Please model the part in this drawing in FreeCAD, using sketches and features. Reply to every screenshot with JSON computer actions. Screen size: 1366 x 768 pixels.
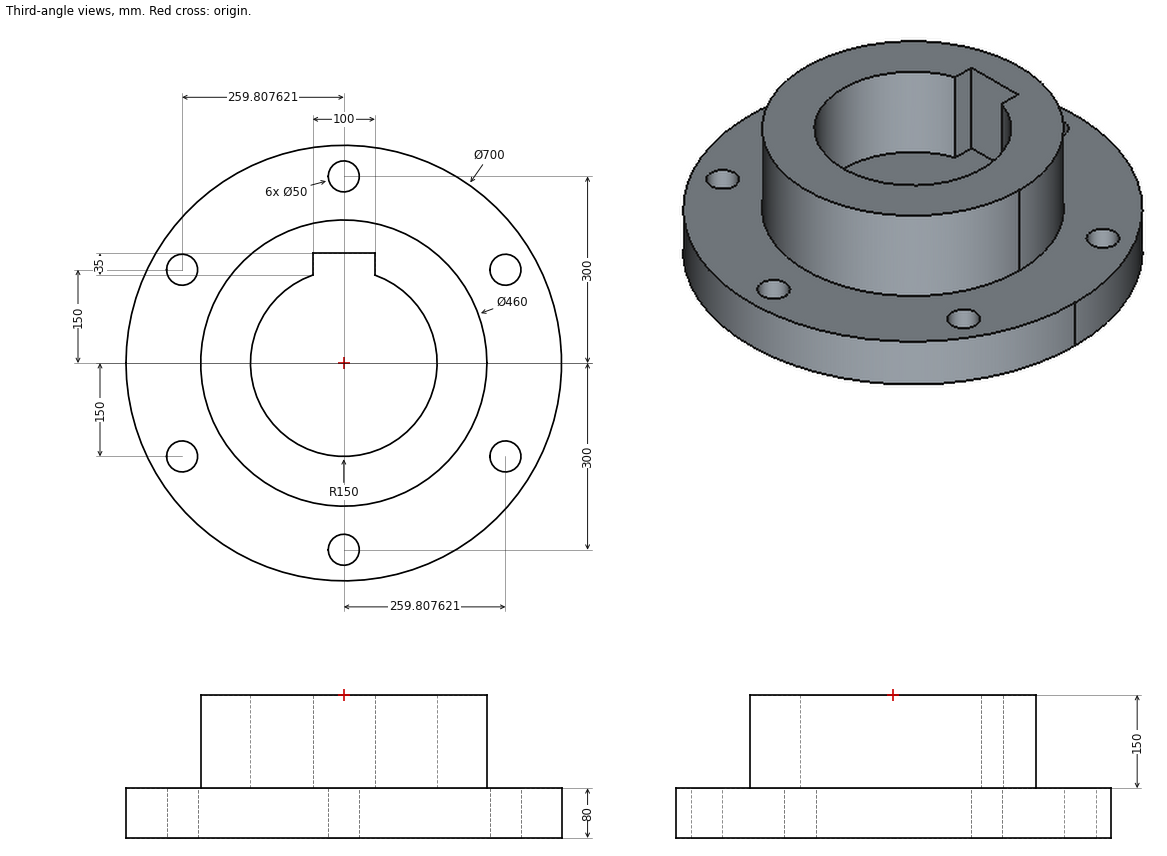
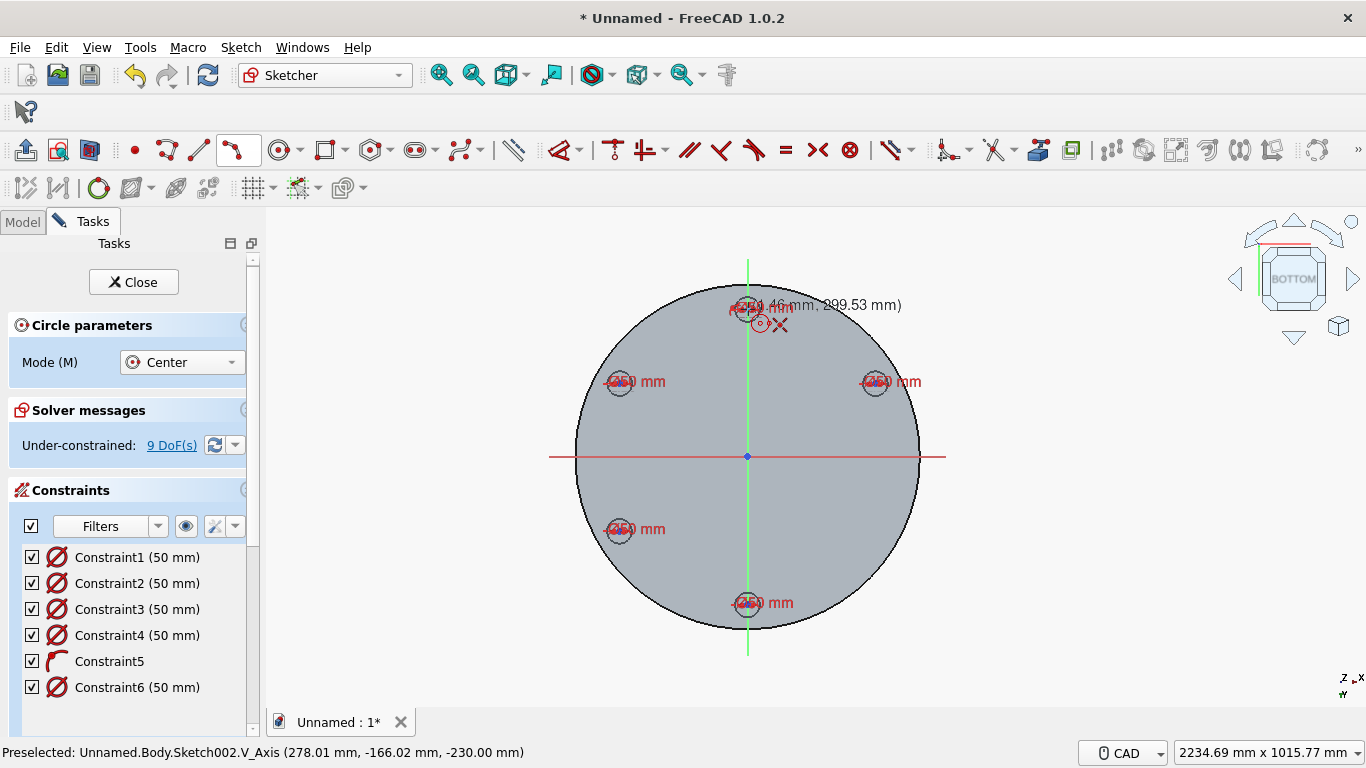
{"action": "scroll", "coordinate": [875, 531], "scroll_direction": "up", "scroll_amount": 4}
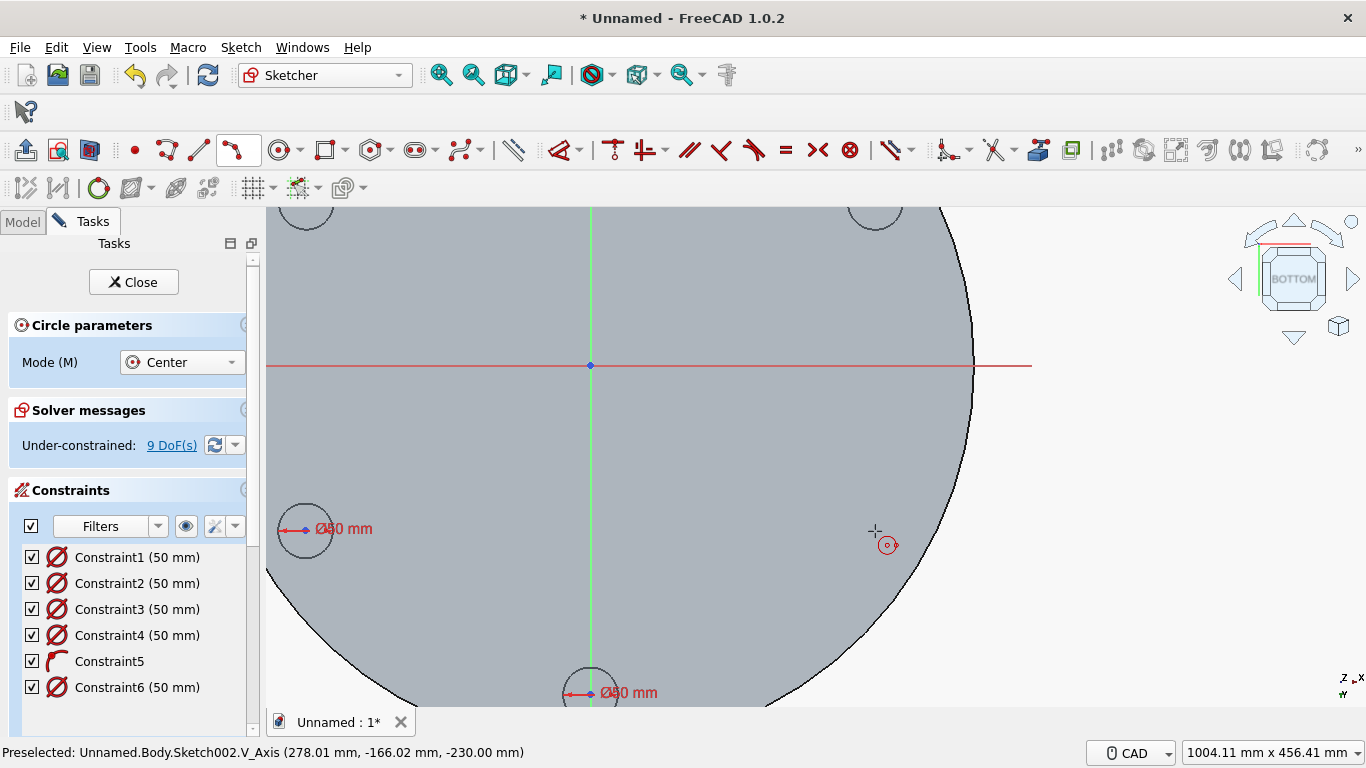
{"action": "left_click", "coordinate": [875, 530]}
{"action": "mouse_move", "coordinate": [895, 510]}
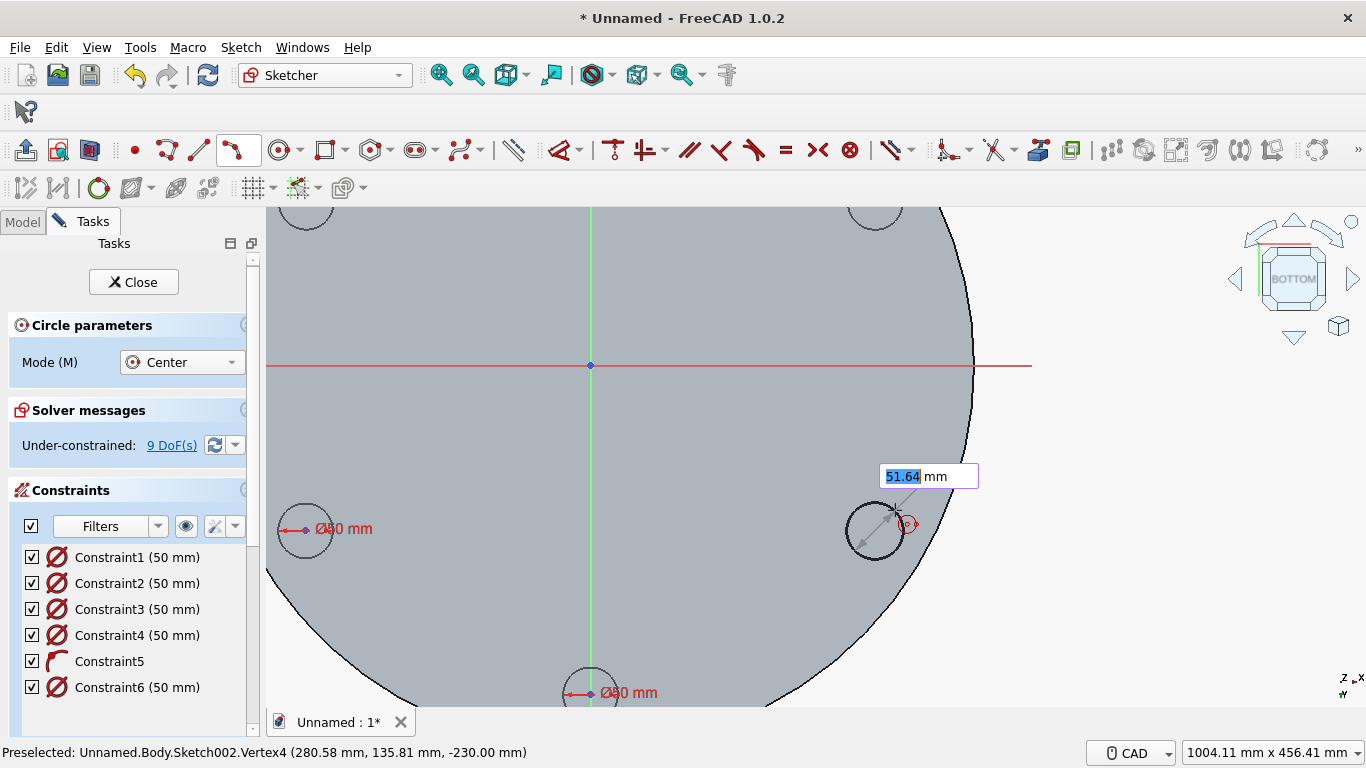
{"action": "type", "text": "50"}
{"action": "key", "text": "Return"}
{"action": "key", "text": "Escape"}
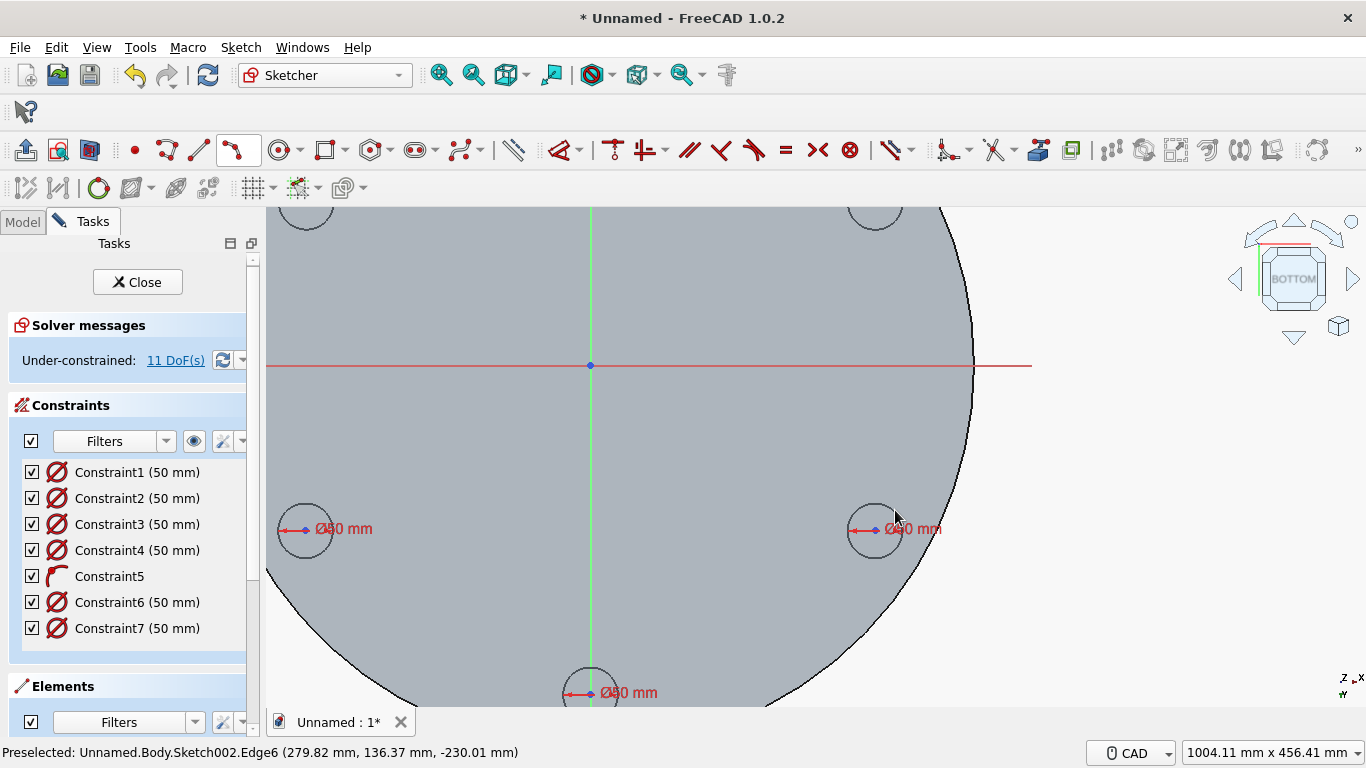
{"action": "scroll", "coordinate": [876, 532], "scroll_direction": "down", "scroll_amount": 4}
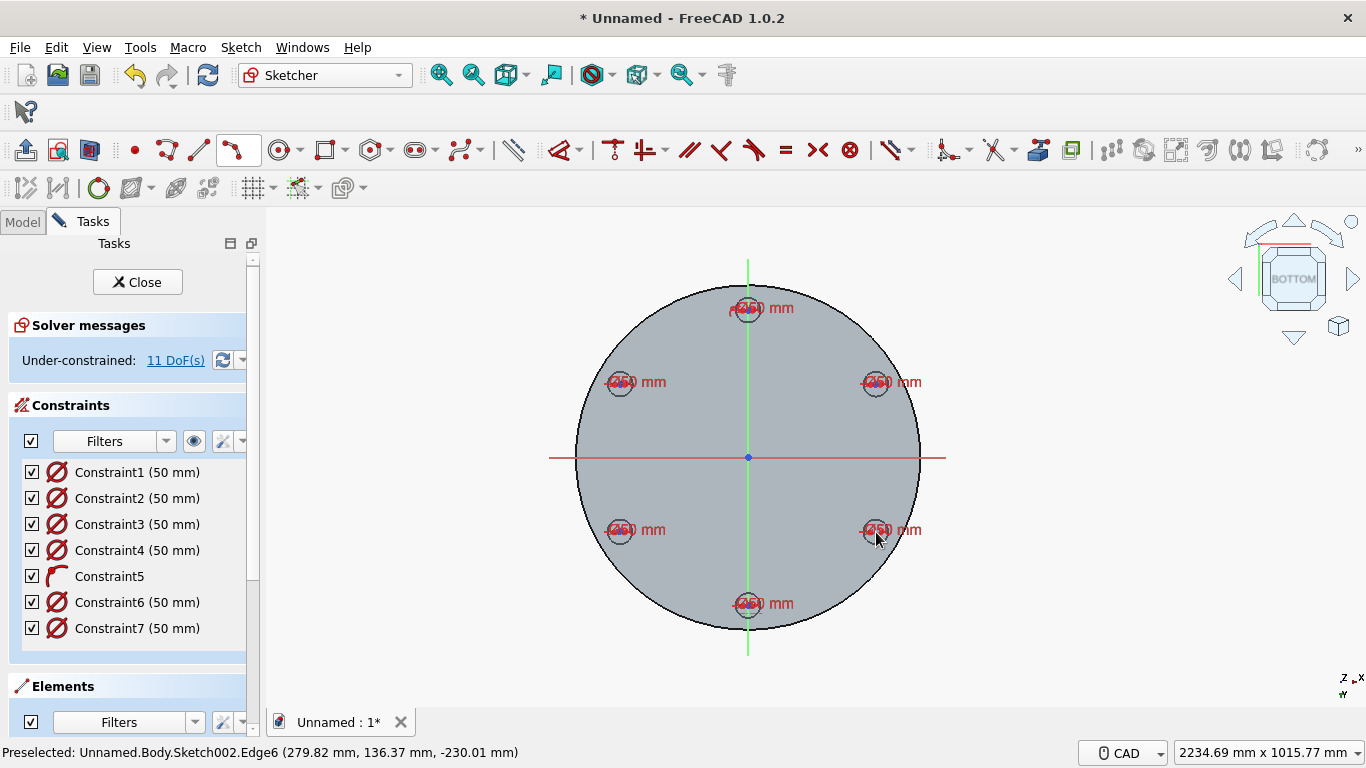
{"action": "left_click", "coordinate": [748, 606]}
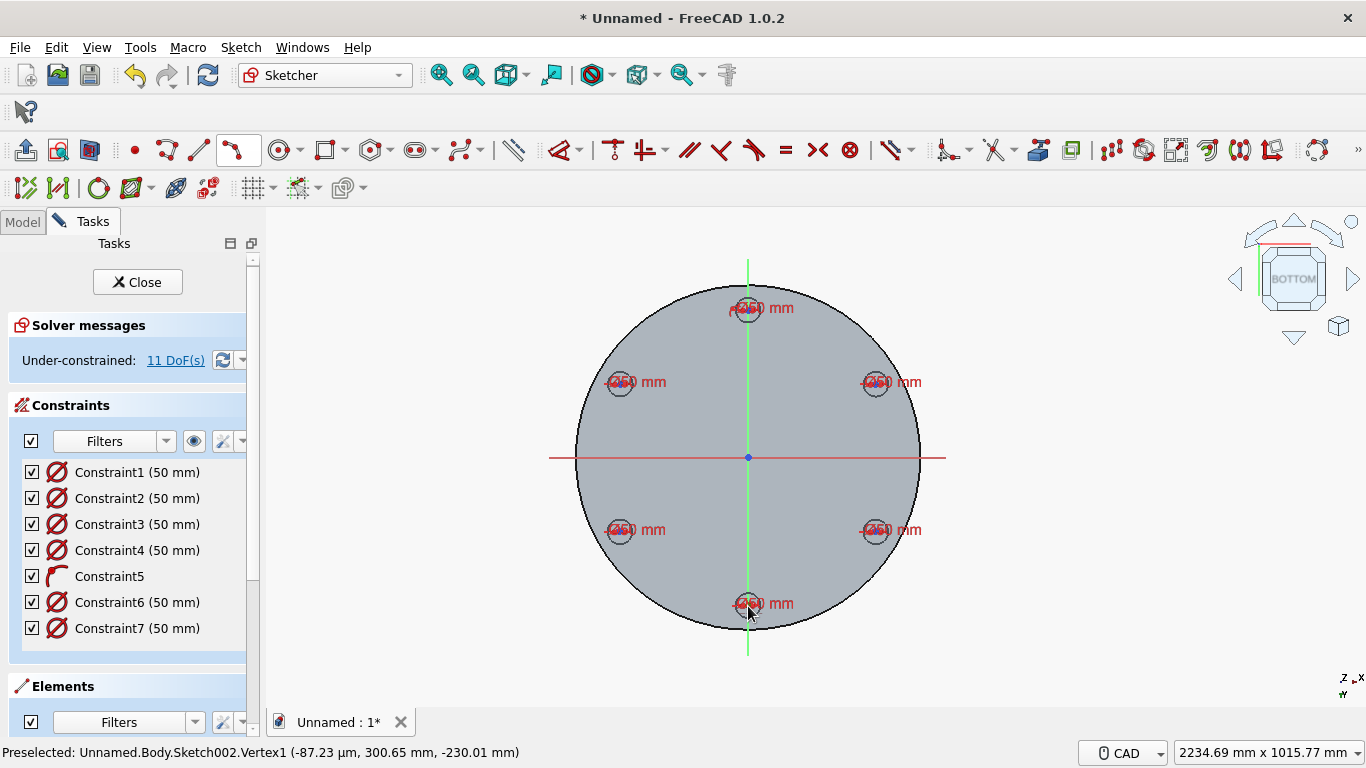
{"action": "left_click", "coordinate": [748, 552]}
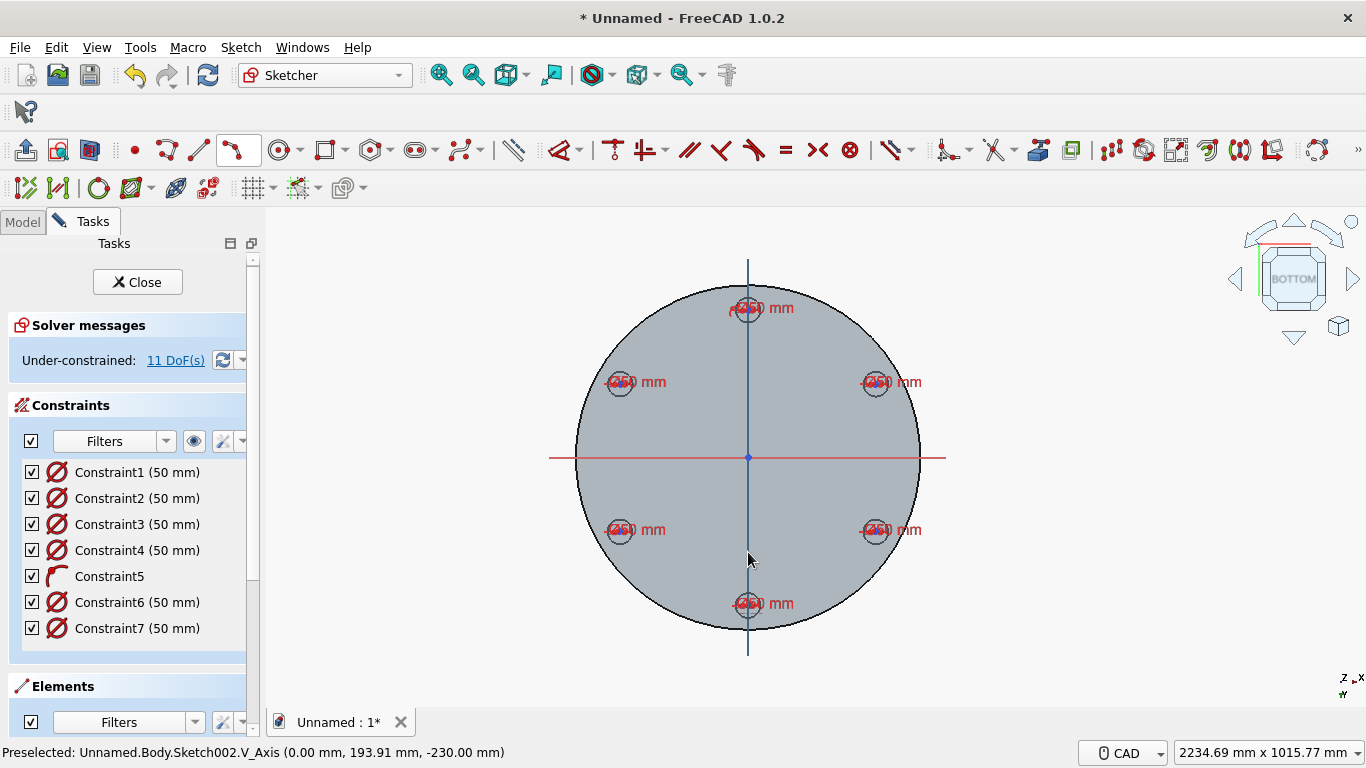
{"action": "key", "text": "c"}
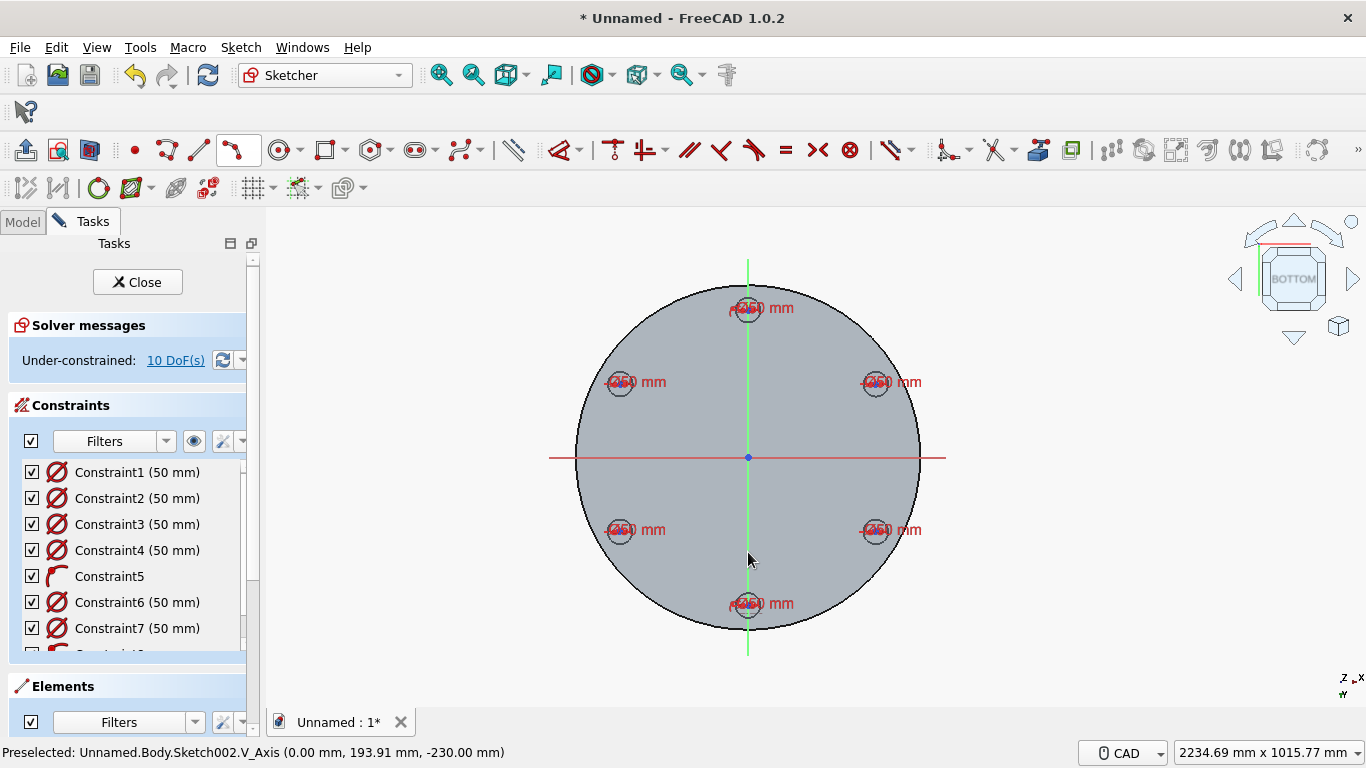
{"action": "left_click", "coordinate": [620, 532]}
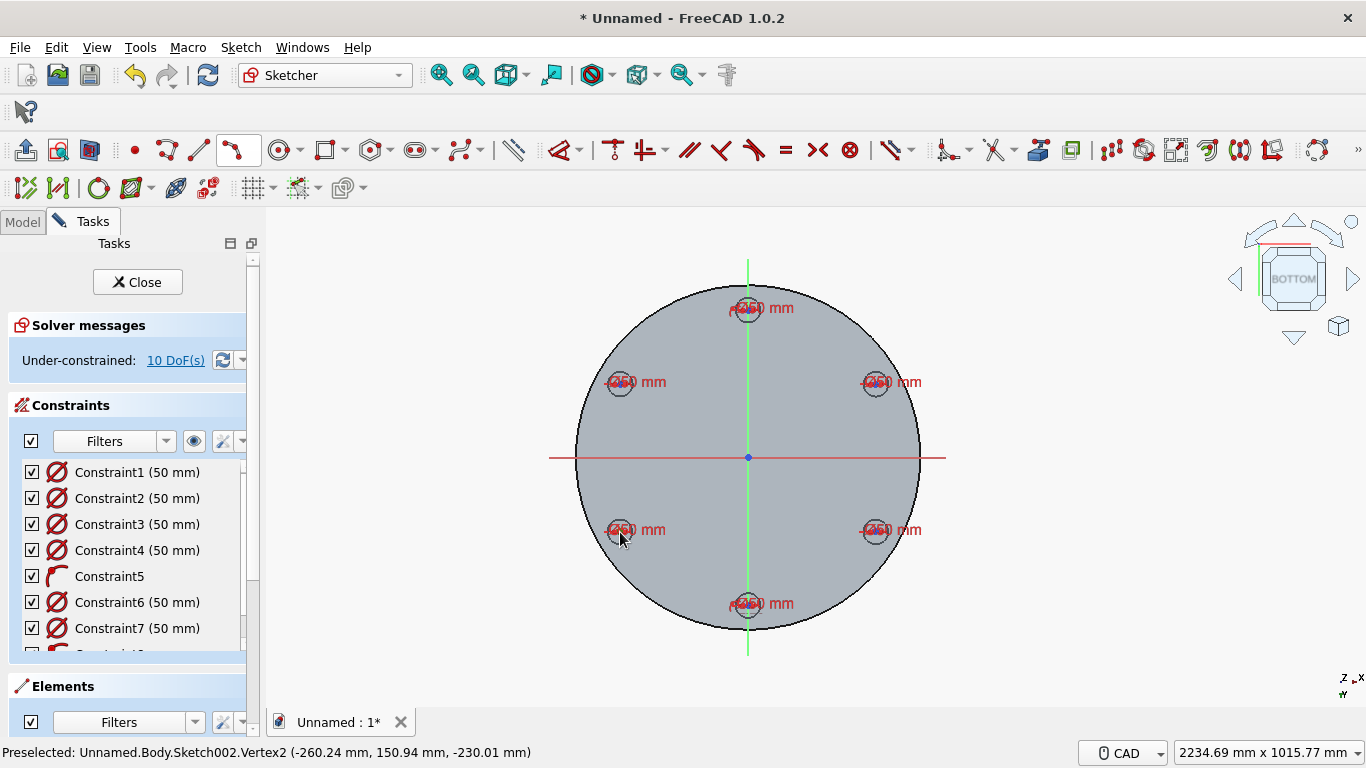
{"action": "left_click", "coordinate": [620, 384]}